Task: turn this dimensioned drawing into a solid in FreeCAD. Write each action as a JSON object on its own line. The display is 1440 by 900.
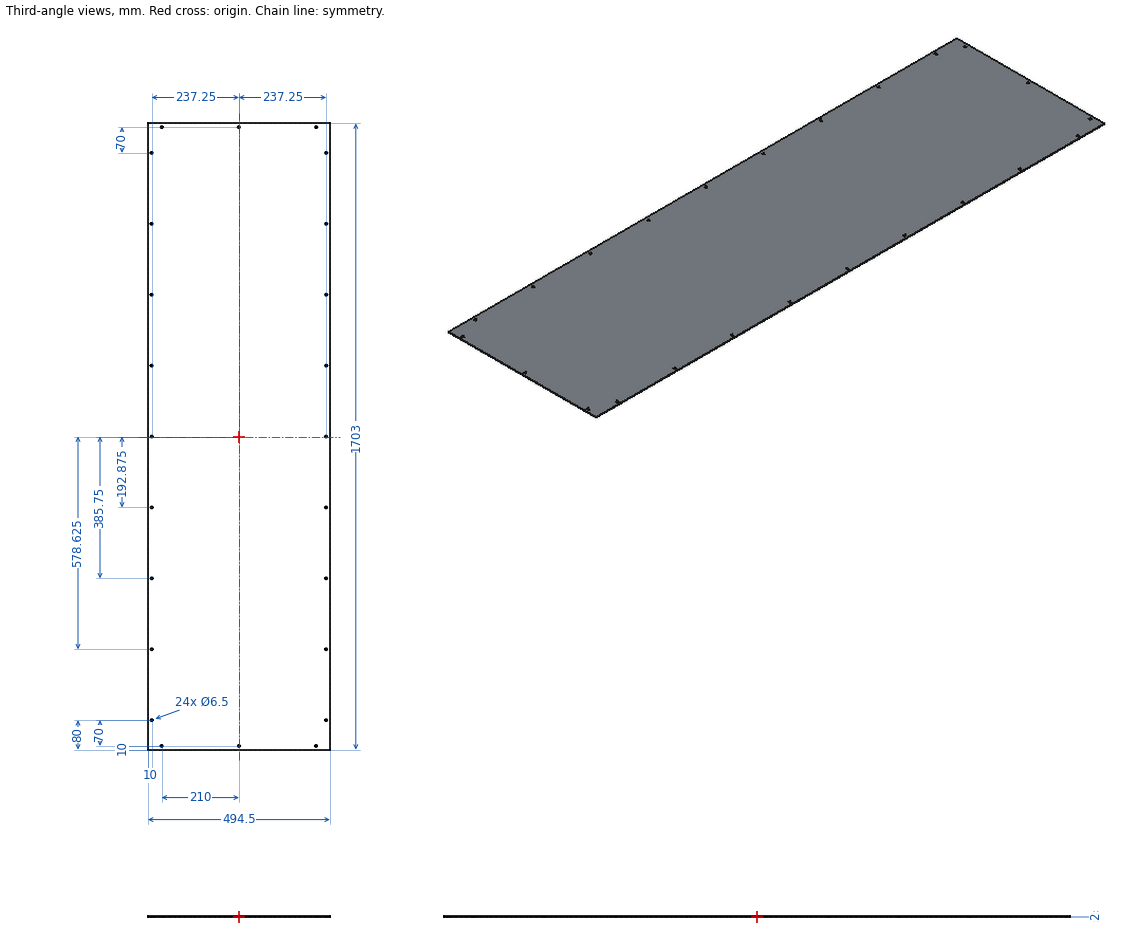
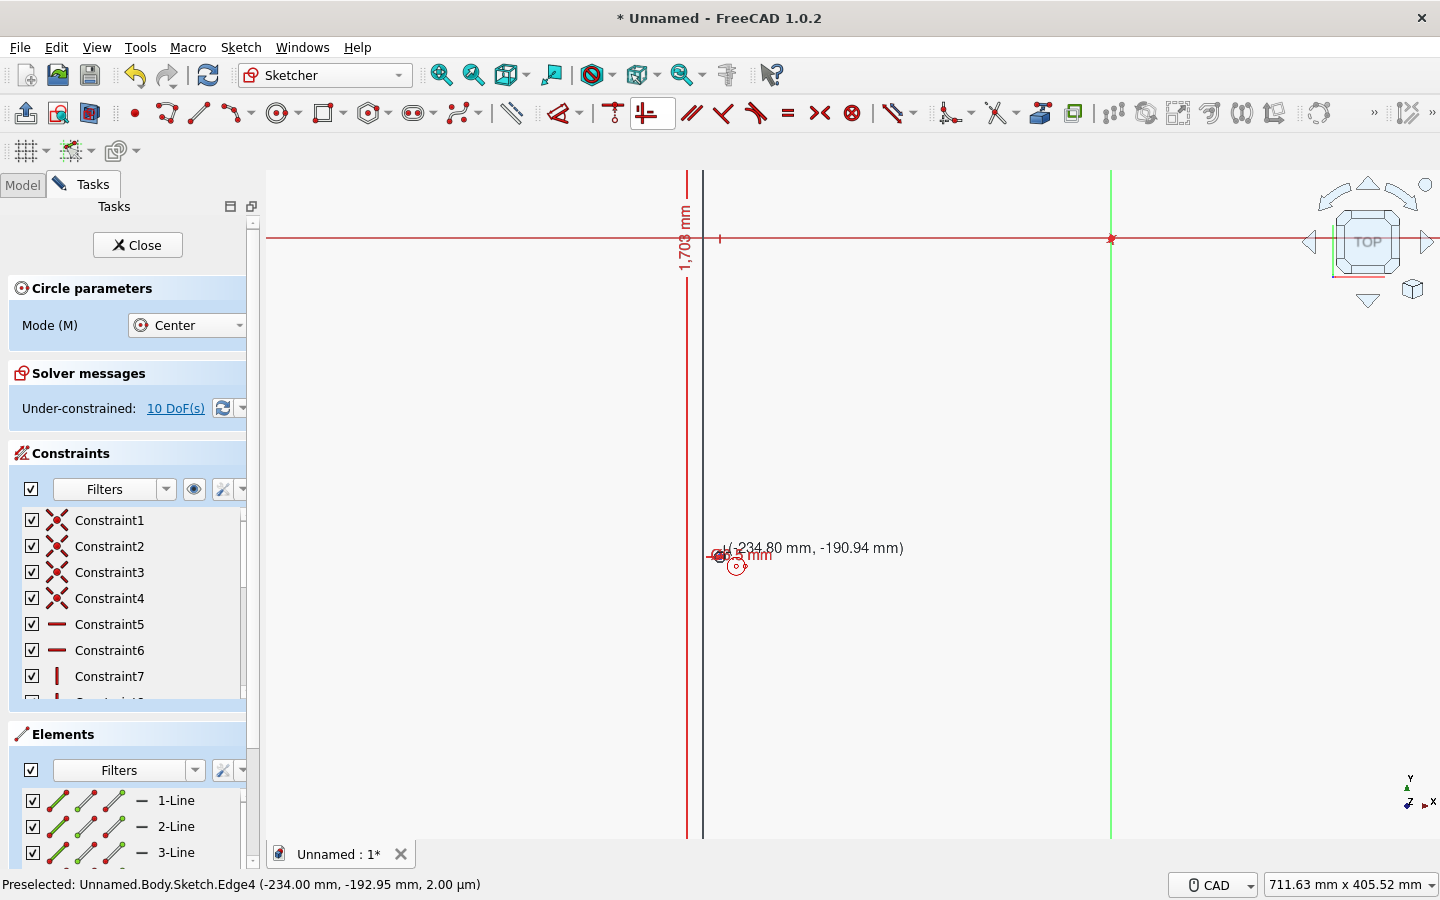
{"action": "scroll", "coordinate": [720, 557], "scroll_direction": "down", "scroll_amount": 9}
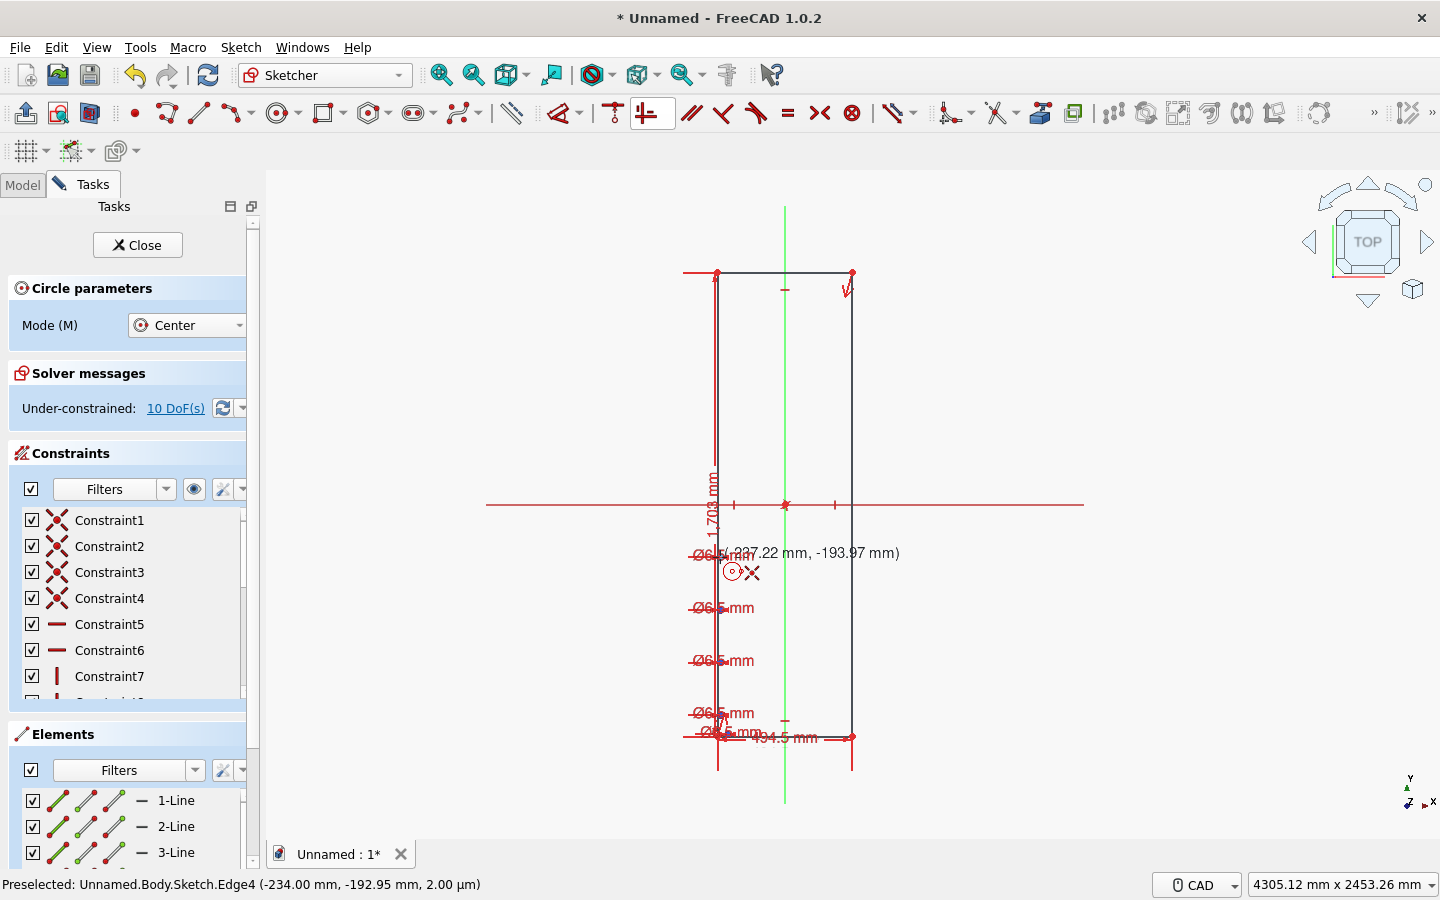
{"action": "scroll", "coordinate": [785, 734], "scroll_direction": "up", "scroll_amount": 17}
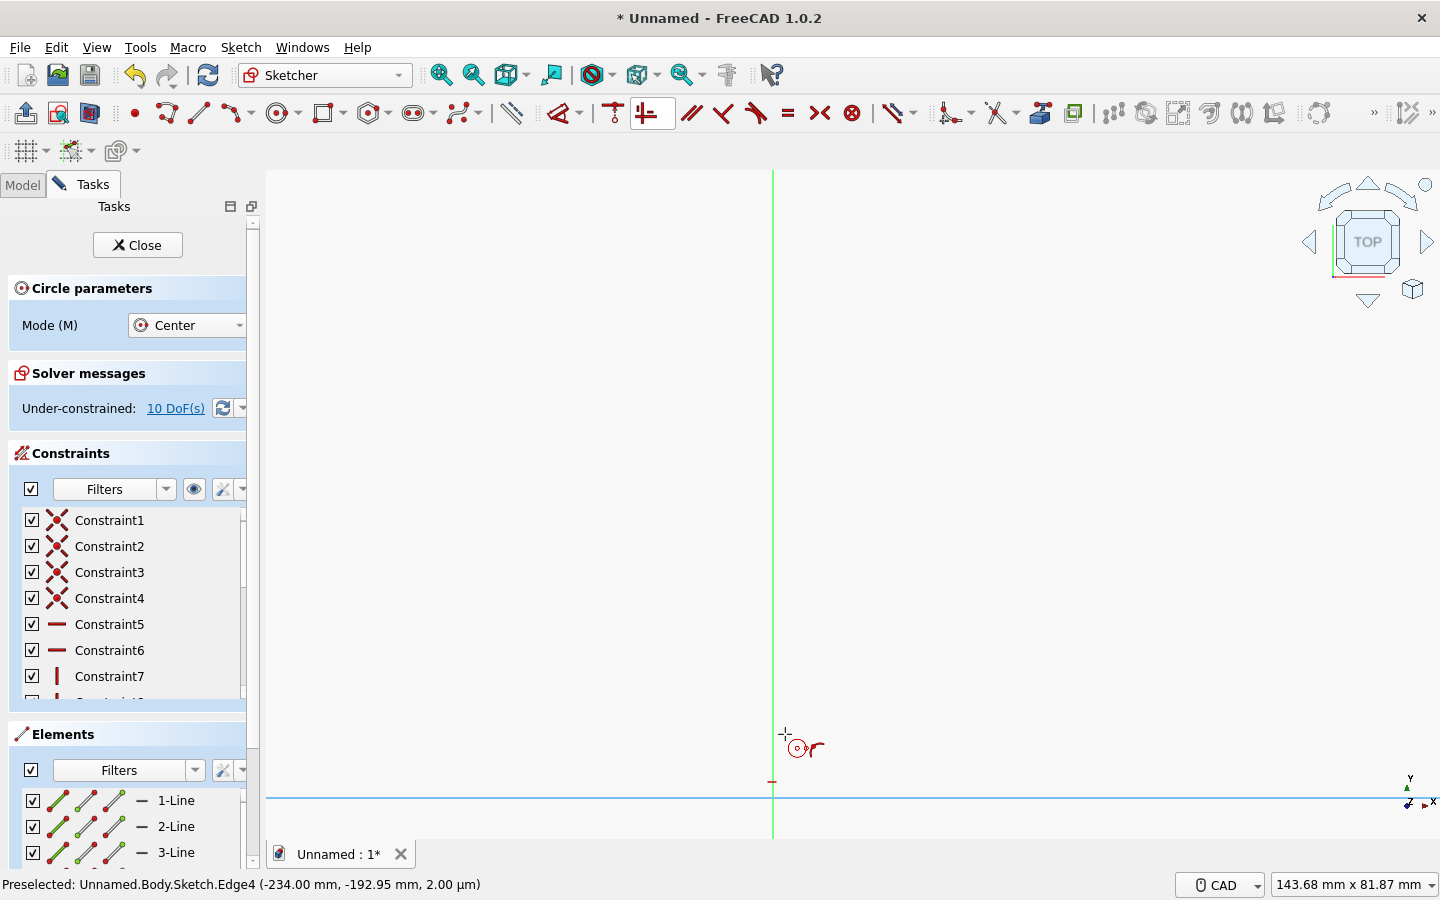
{"action": "scroll", "coordinate": [785, 735], "scroll_direction": "down", "scroll_amount": 17}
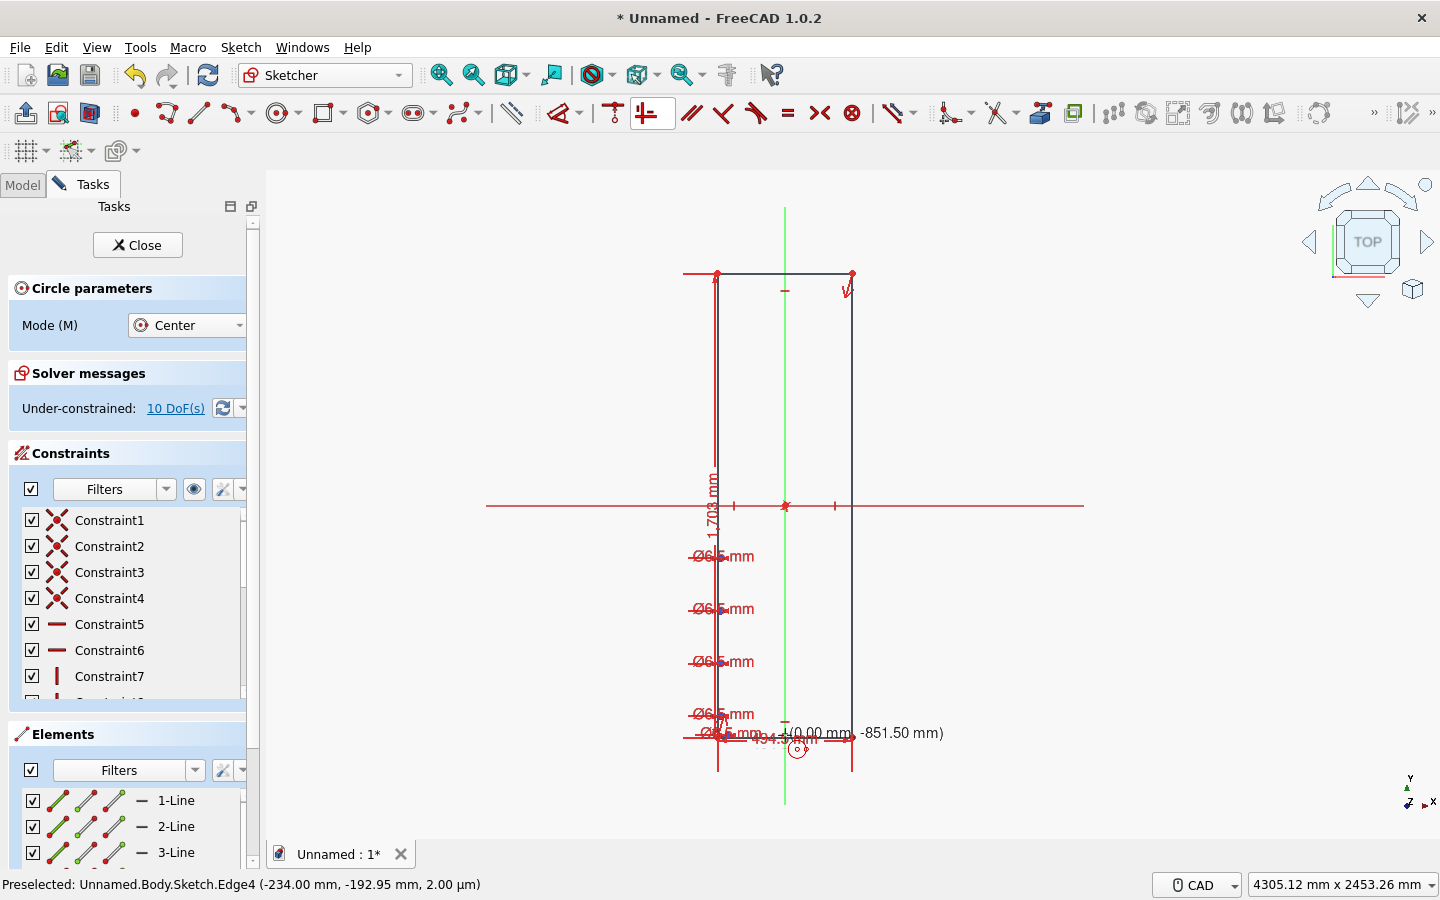
{"action": "scroll", "coordinate": [785, 735], "scroll_direction": "up", "scroll_amount": 9}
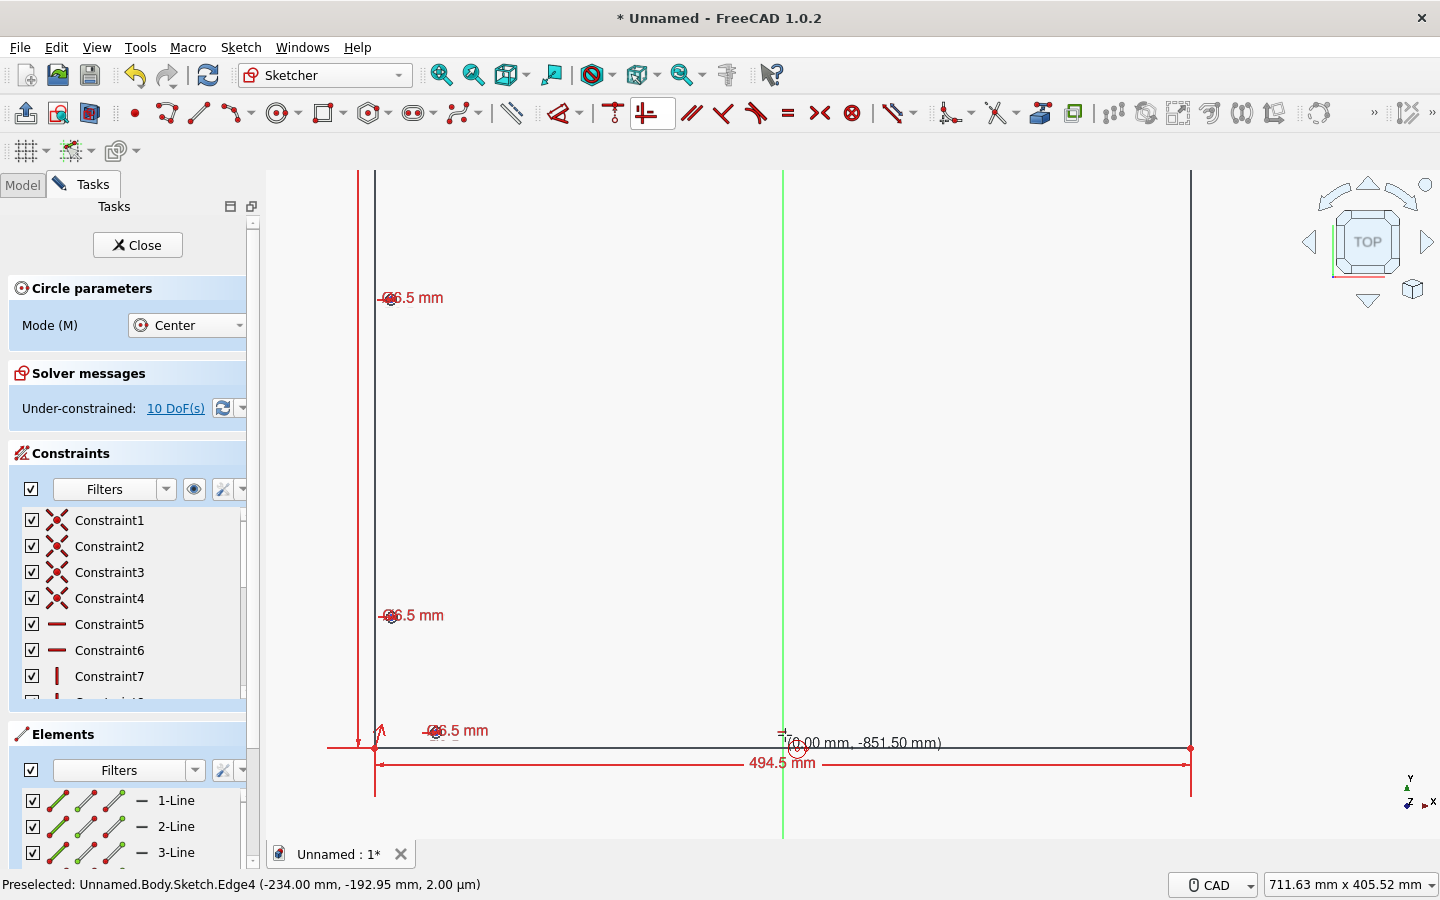
{"action": "left_click", "coordinate": [783, 732]}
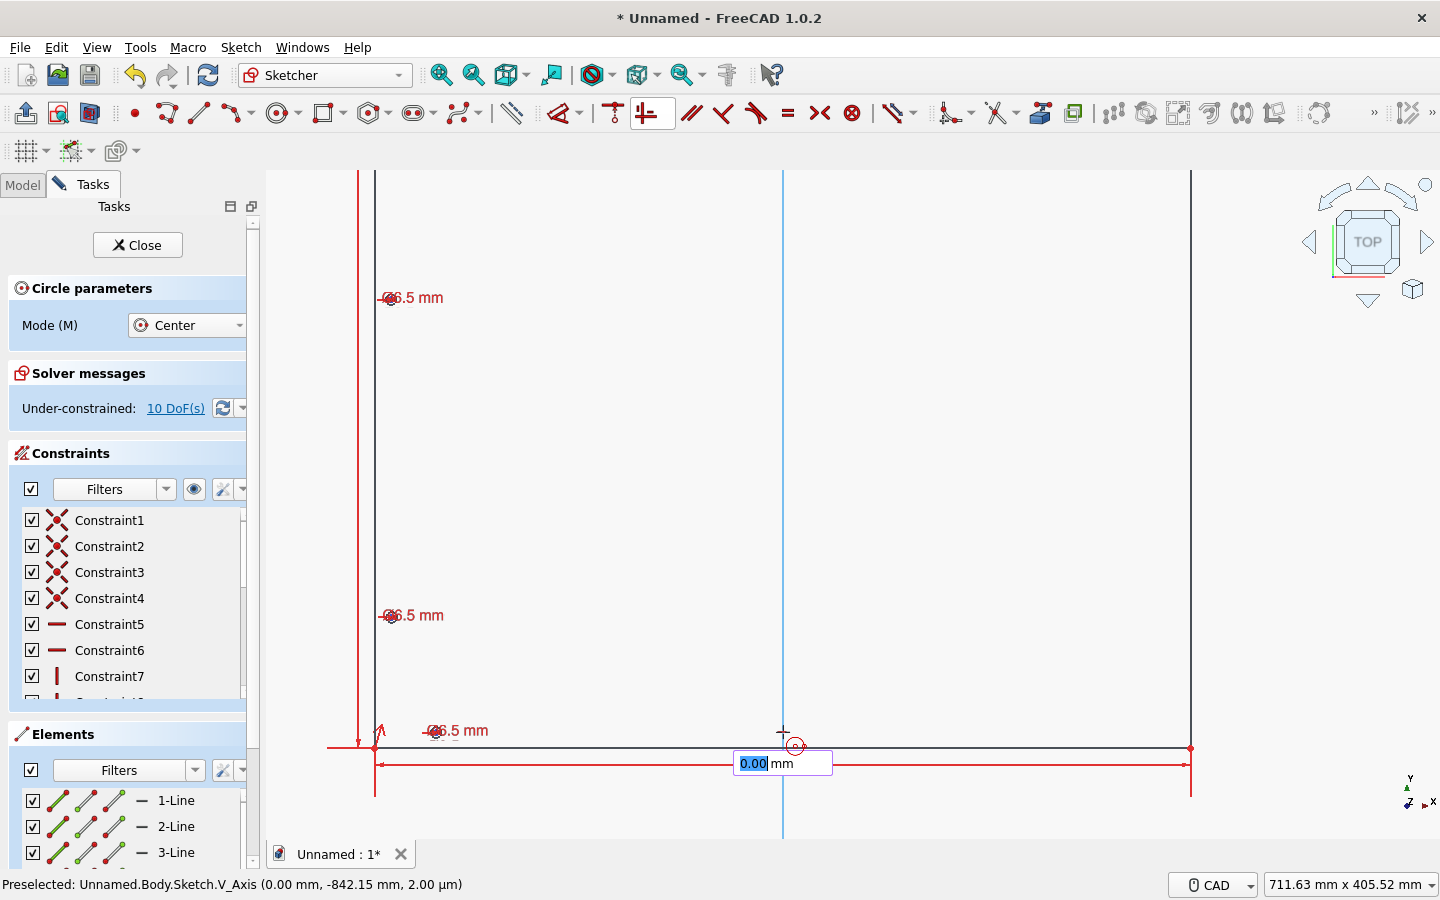
{"action": "scroll", "coordinate": [788, 730], "scroll_direction": "up", "scroll_amount": 6}
{"action": "mouse_move", "coordinate": [787, 728]}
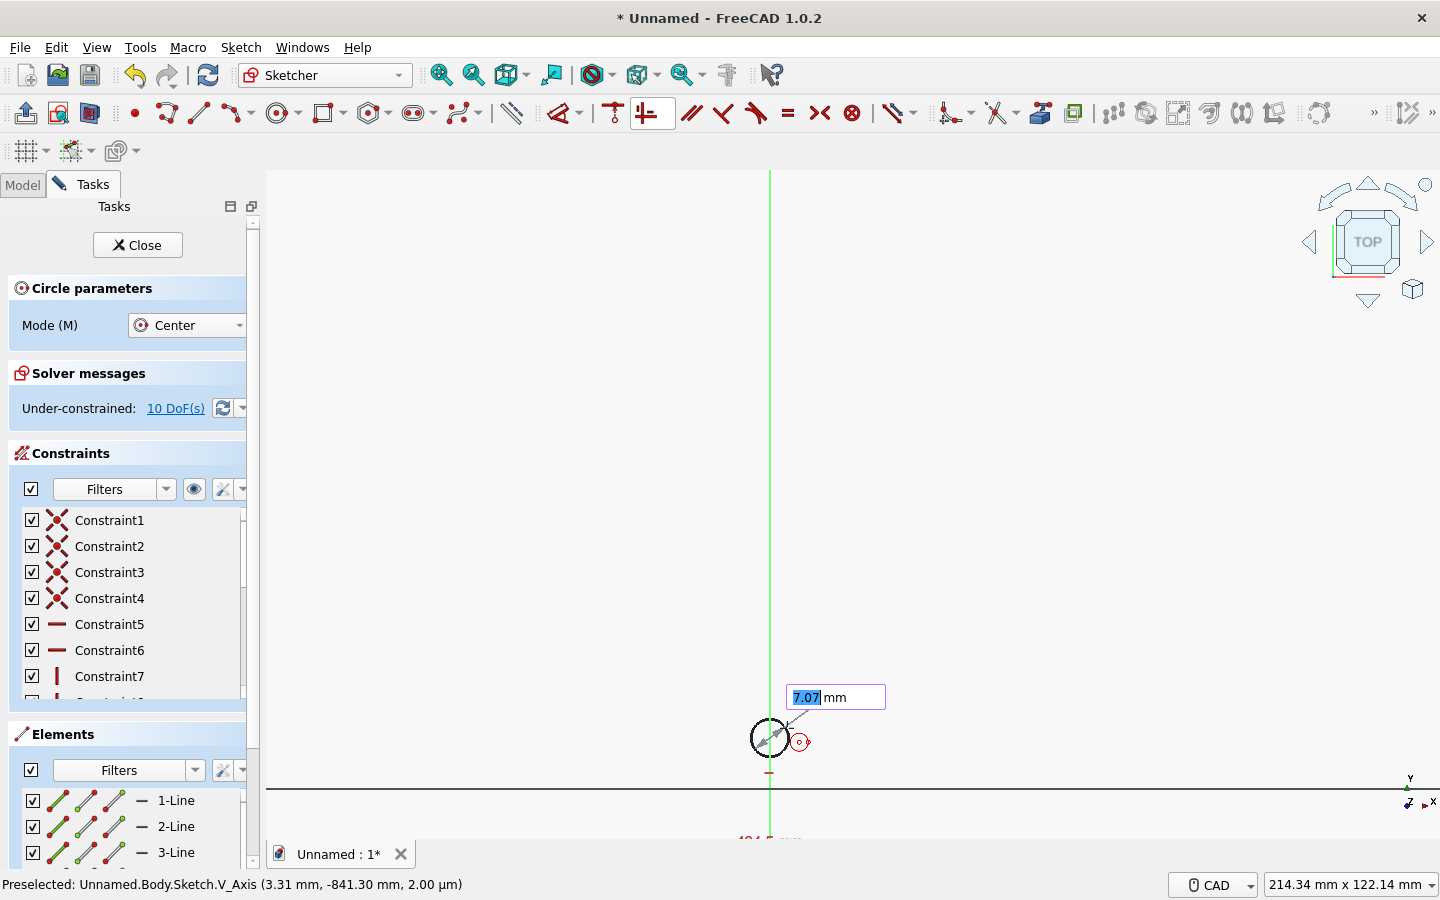
{"action": "type", "text": "6.5"}
{"action": "key", "text": "Return"}